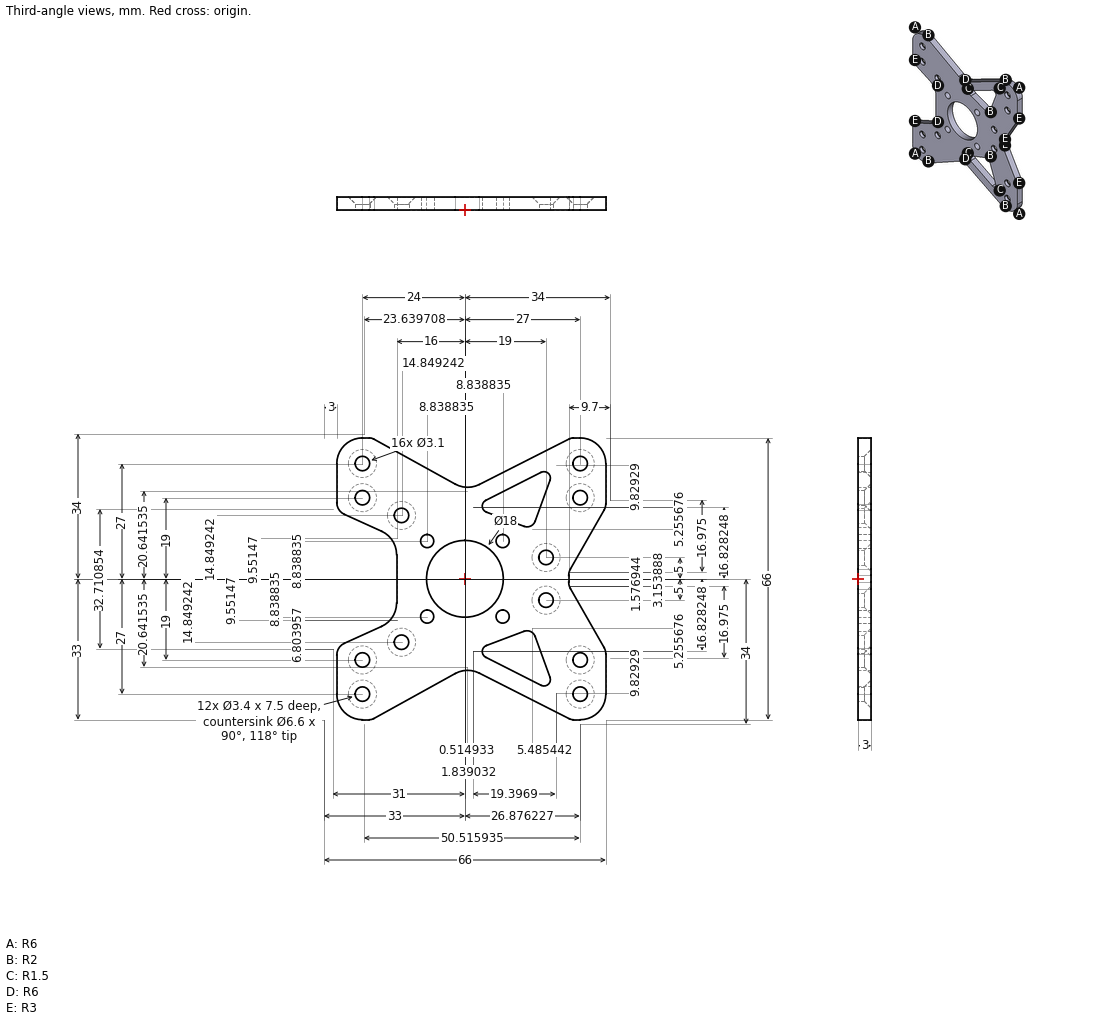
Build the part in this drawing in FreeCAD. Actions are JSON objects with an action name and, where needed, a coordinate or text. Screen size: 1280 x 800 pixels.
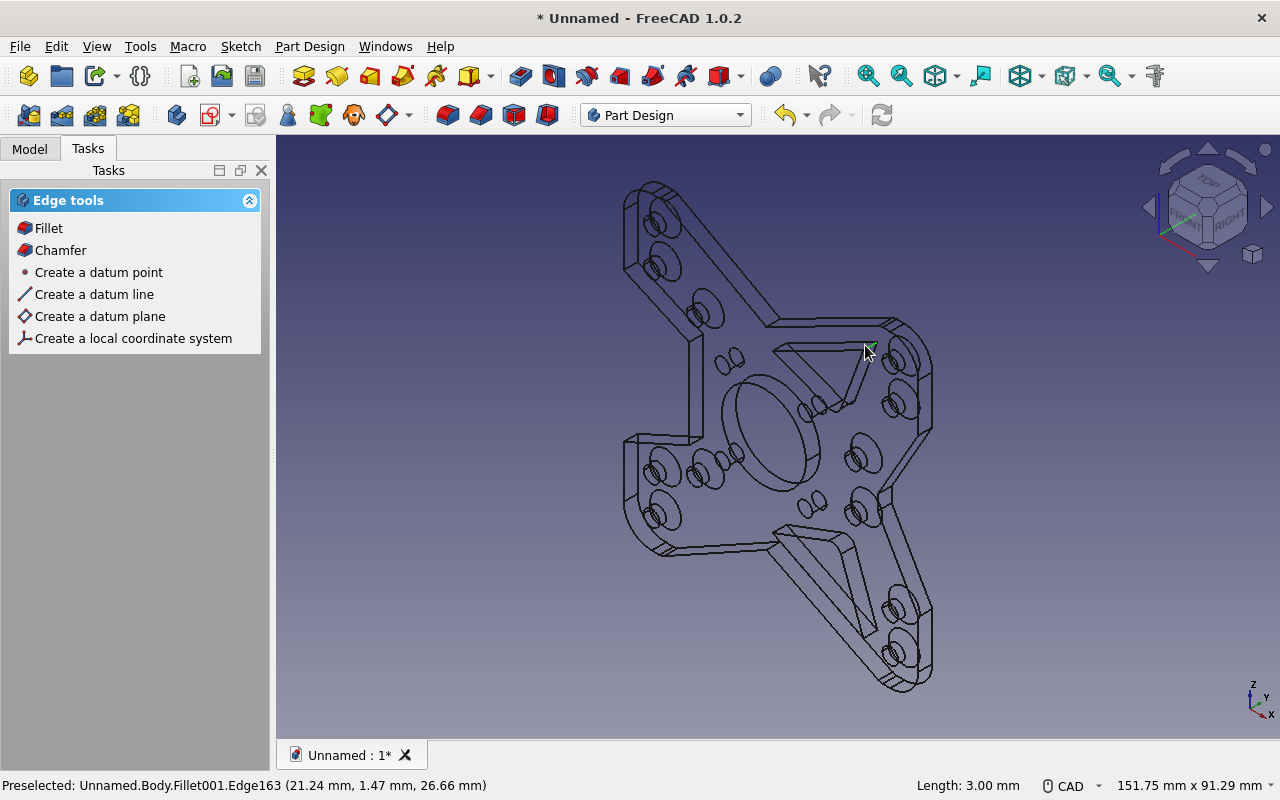
{"action": "left_click", "coordinate": [870, 633], "text": "ctrl"}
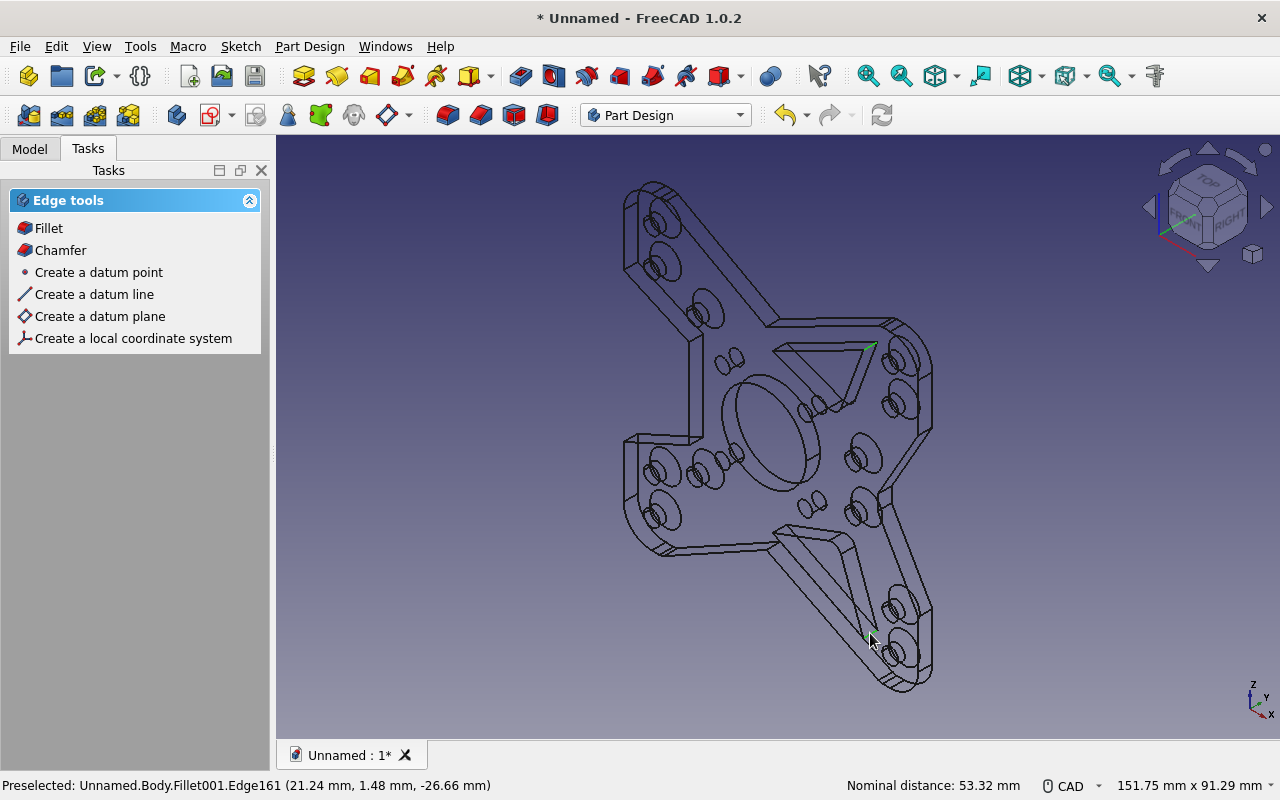
{"action": "left_click", "coordinate": [782, 526], "text": "ctrl"}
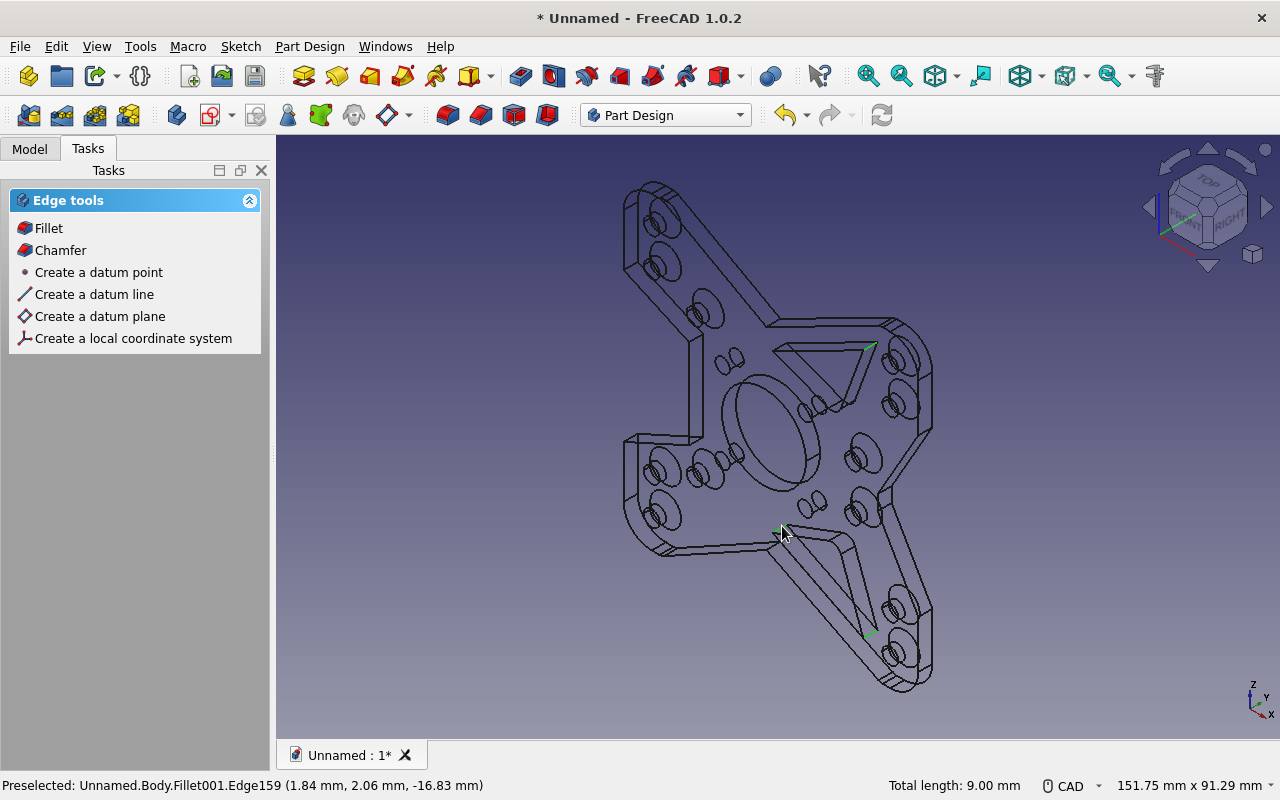
{"action": "scroll", "coordinate": [780, 346], "scroll_direction": "up", "scroll_amount": 6}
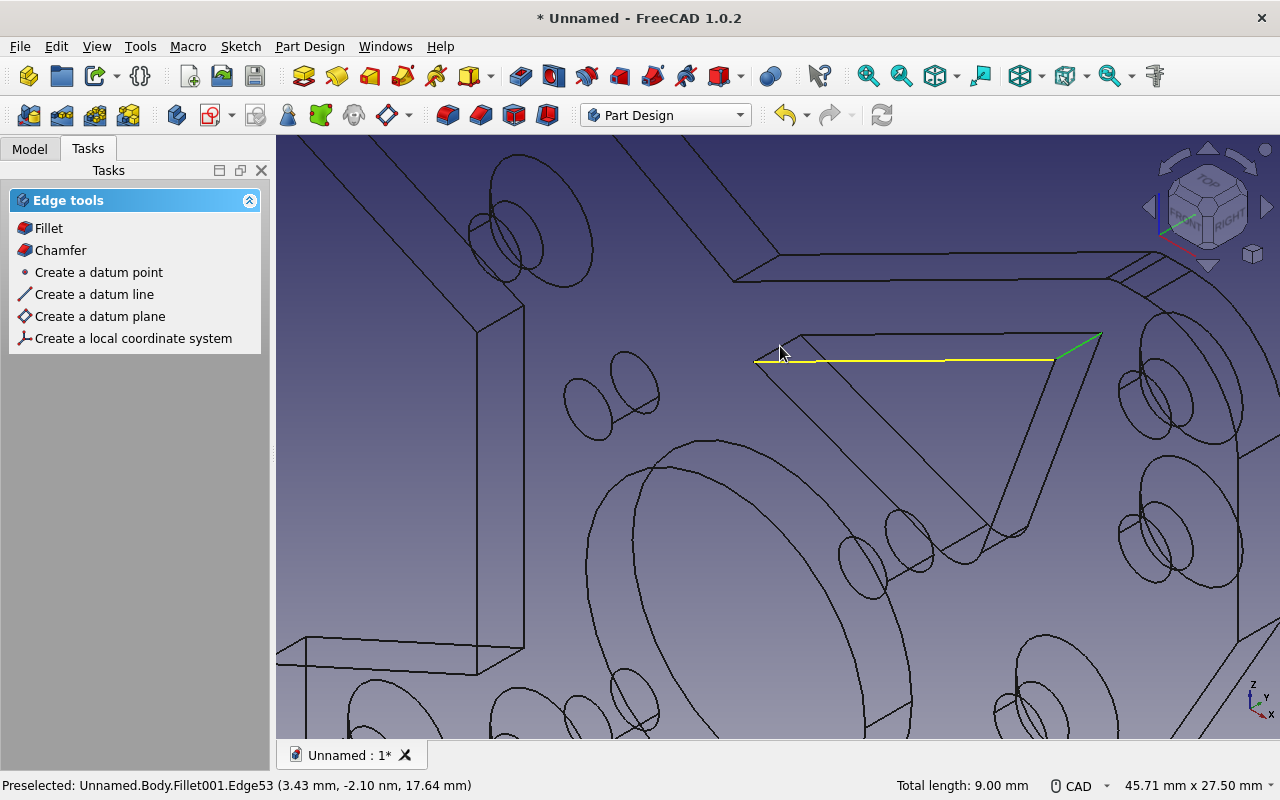
{"action": "left_click", "coordinate": [777, 348], "text": "ctrl"}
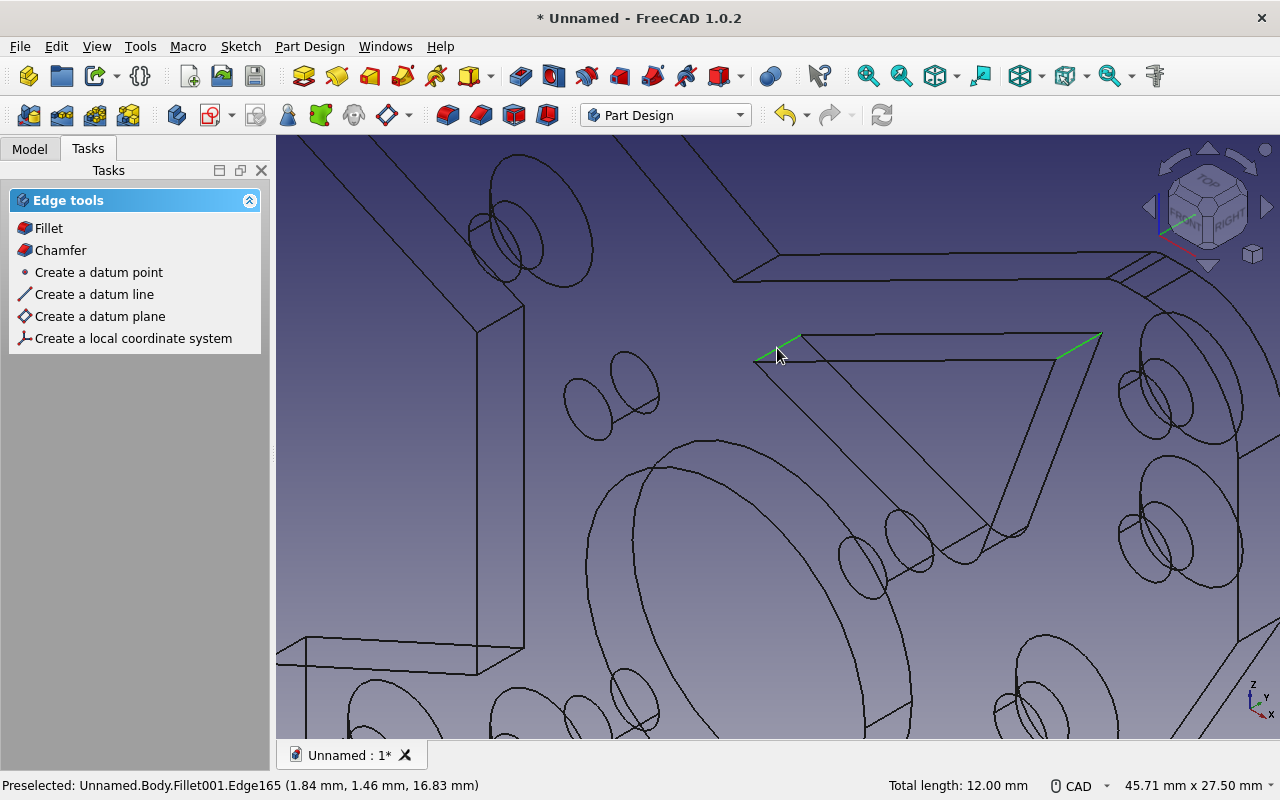
{"action": "key", "text": "v 1"}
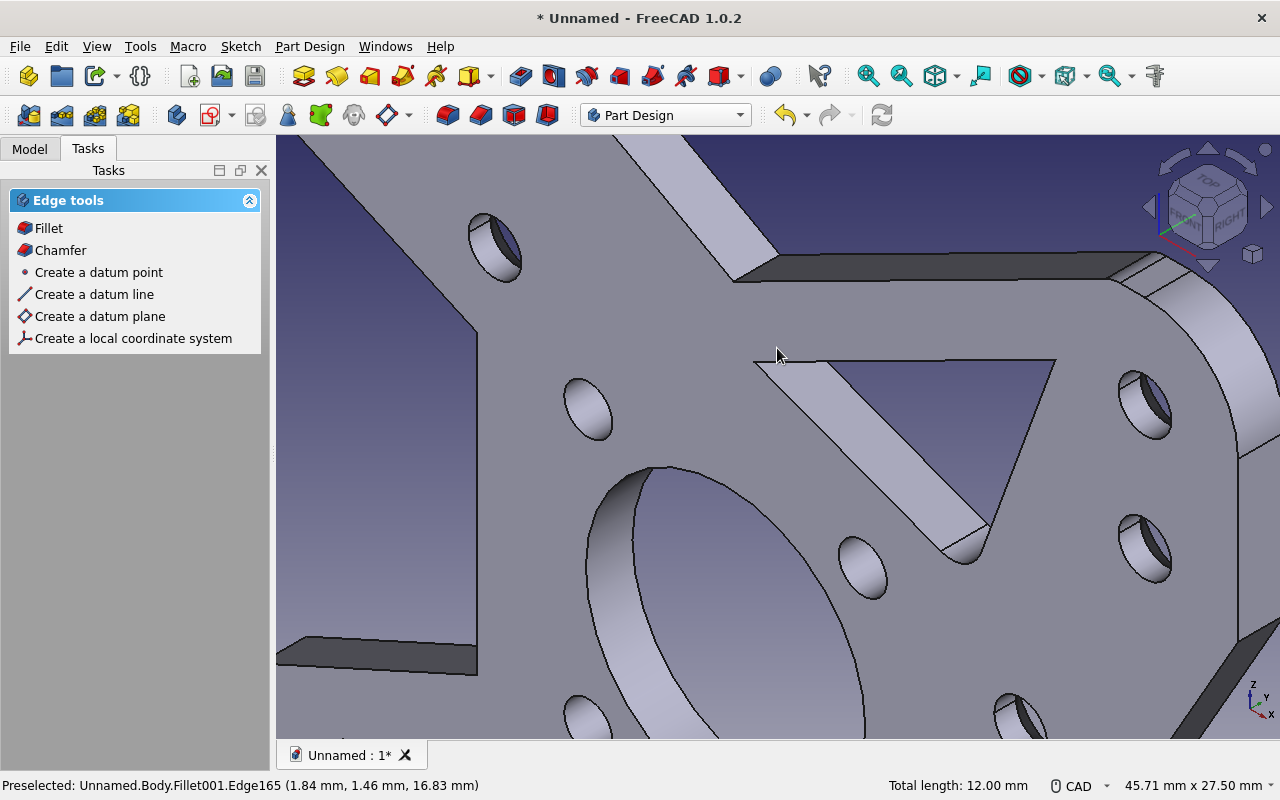
{"action": "left_click", "coordinate": [448, 116]}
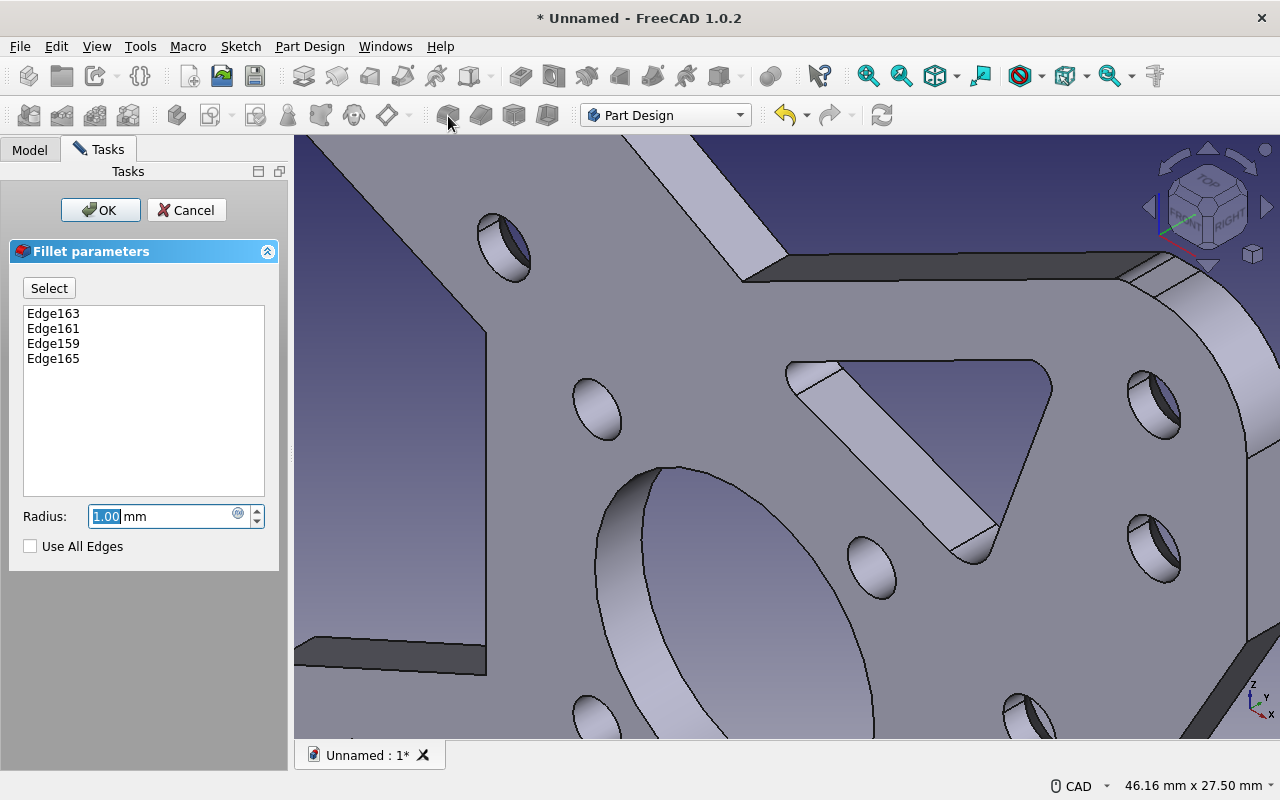
{"action": "type", "text": "1.5"}
{"action": "key", "text": "Tab"}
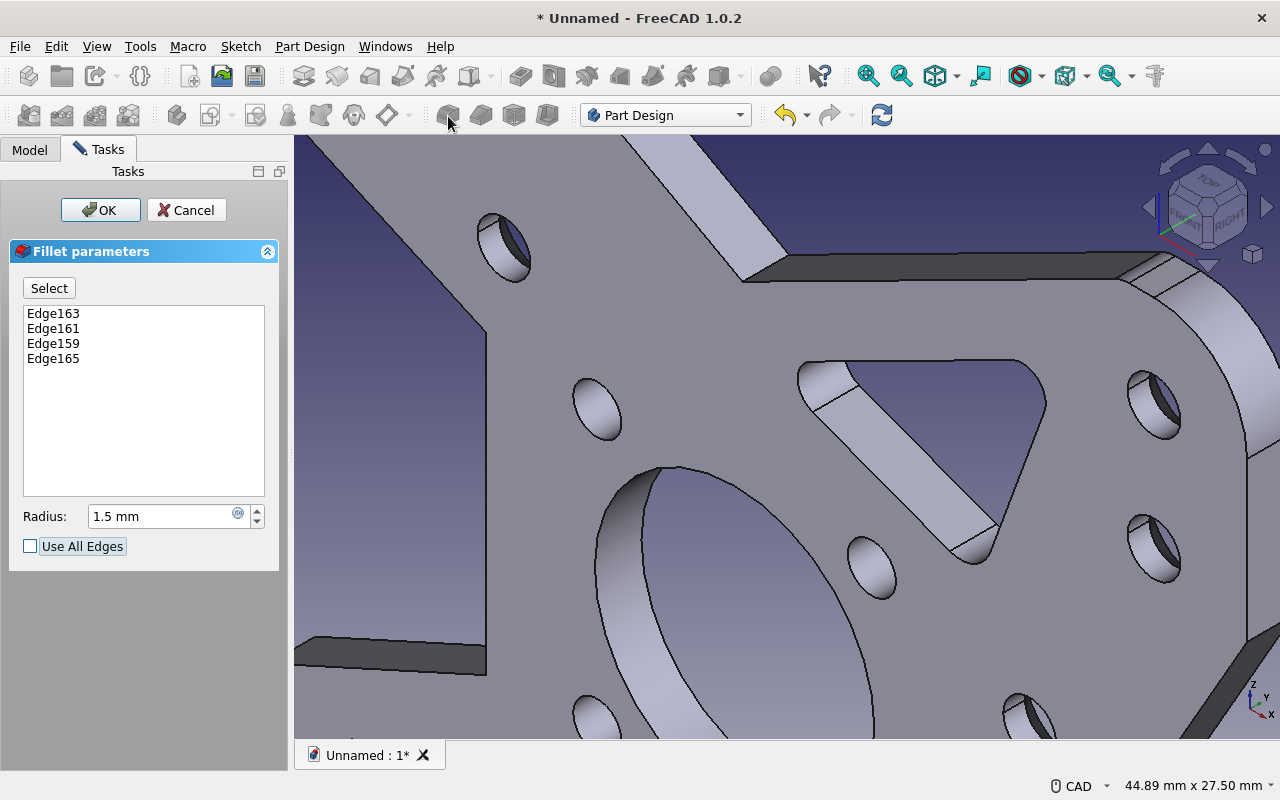
{"action": "left_click", "coordinate": [101, 210]}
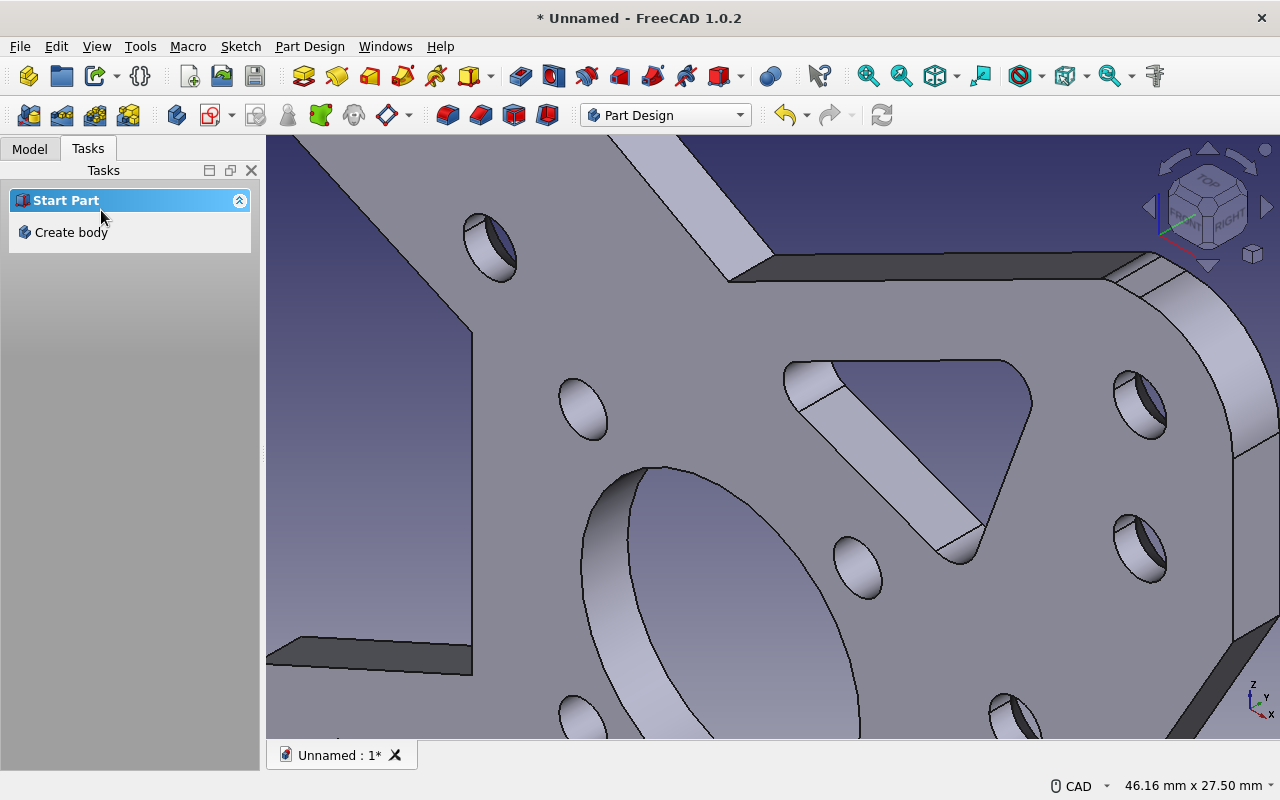
{"action": "left_click", "coordinate": [869, 76]}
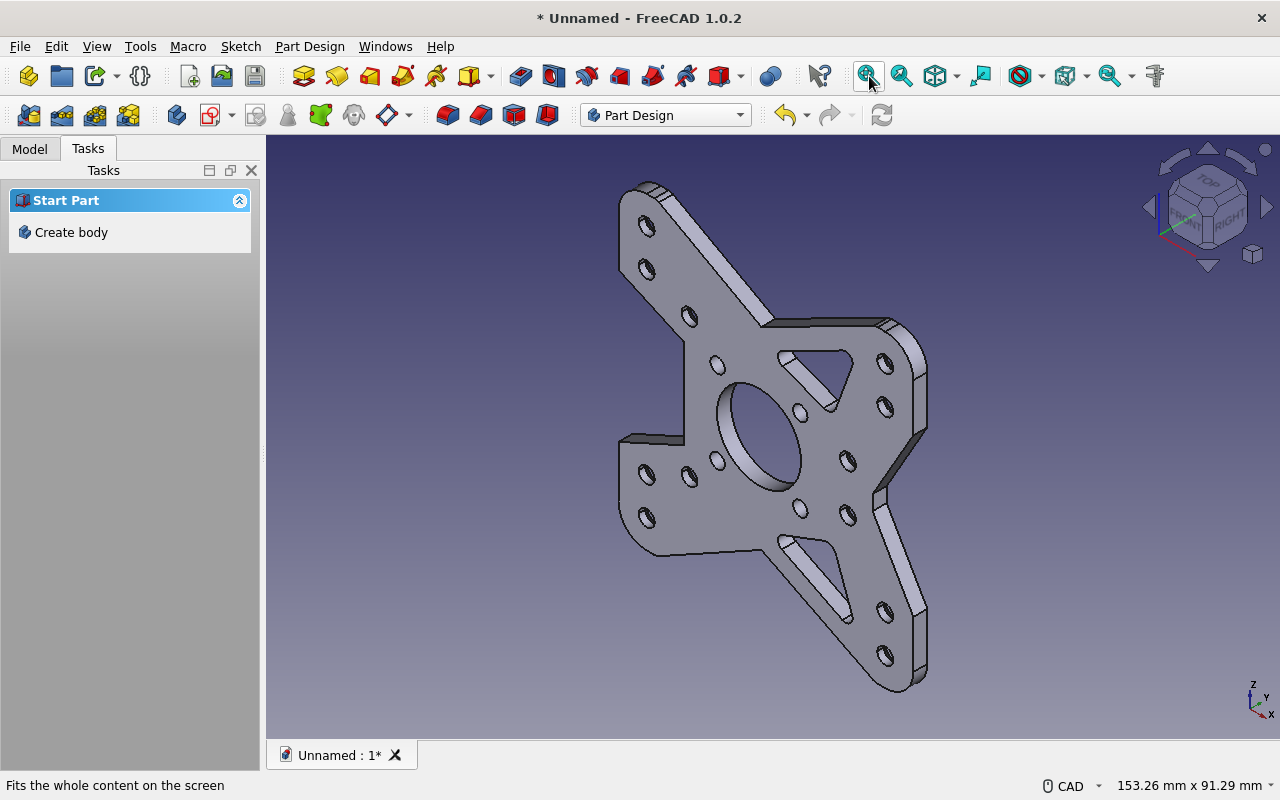
{"action": "scroll", "coordinate": [768, 545], "scroll_direction": "up", "scroll_amount": 4}